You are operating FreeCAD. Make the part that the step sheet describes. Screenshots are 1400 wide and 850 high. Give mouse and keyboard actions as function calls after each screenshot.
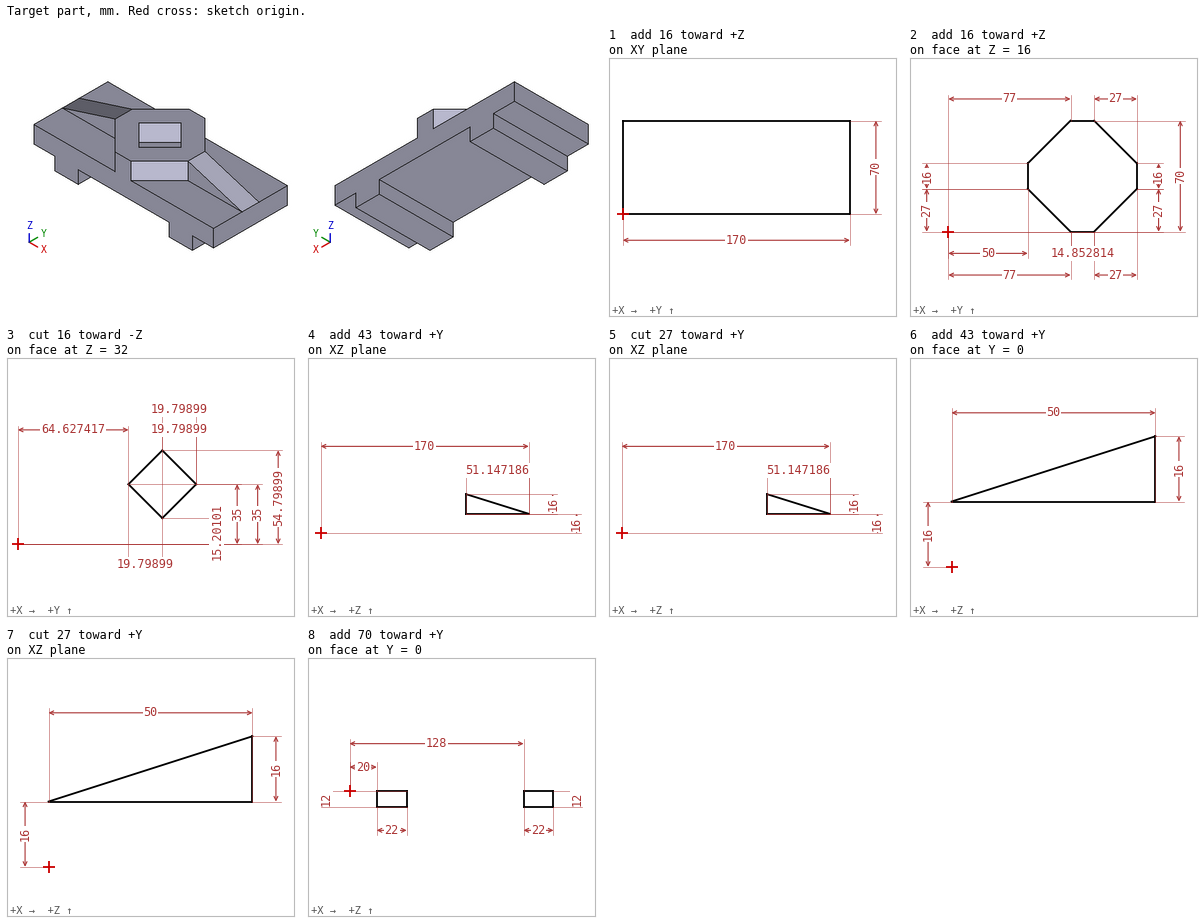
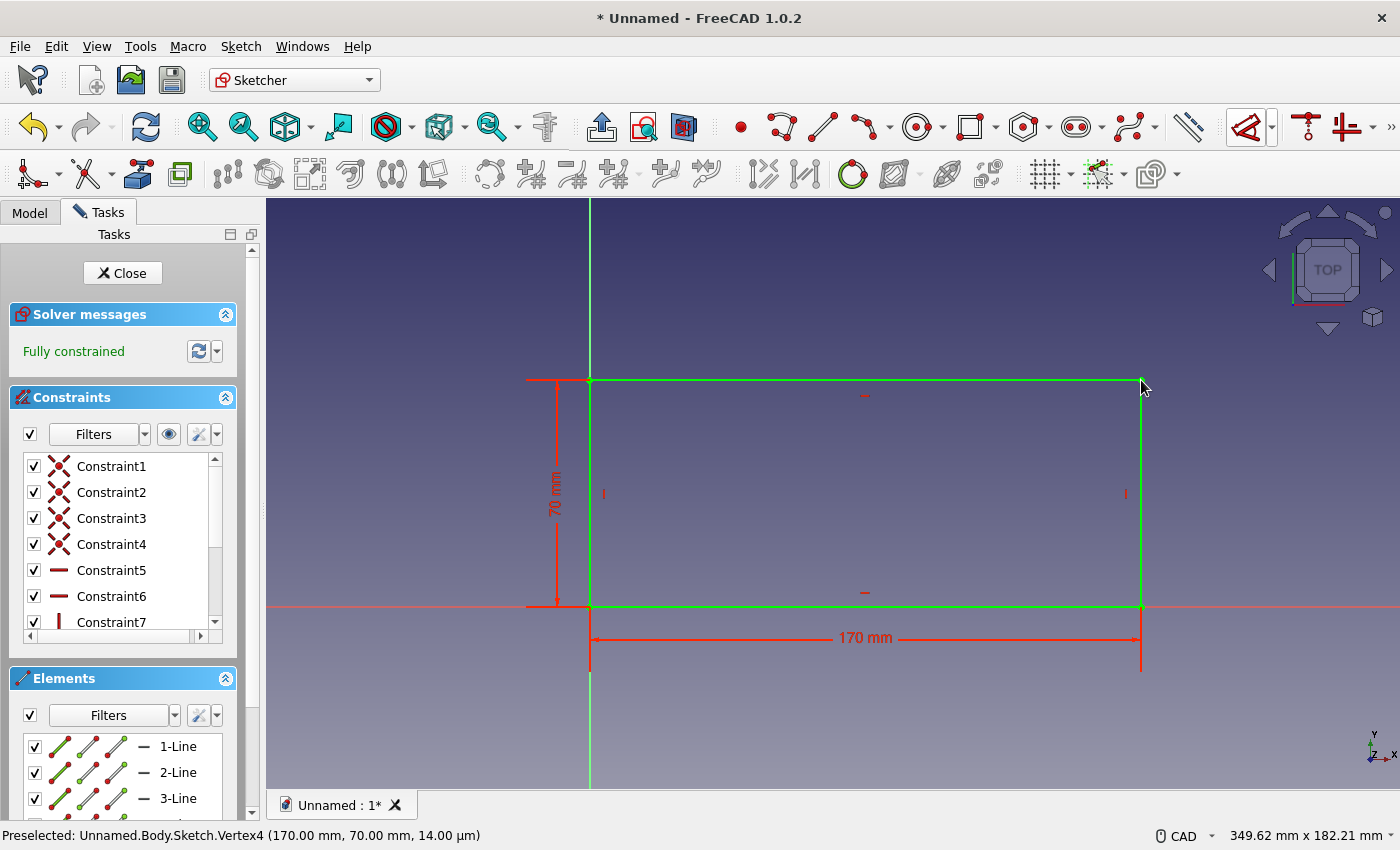
click(123, 273)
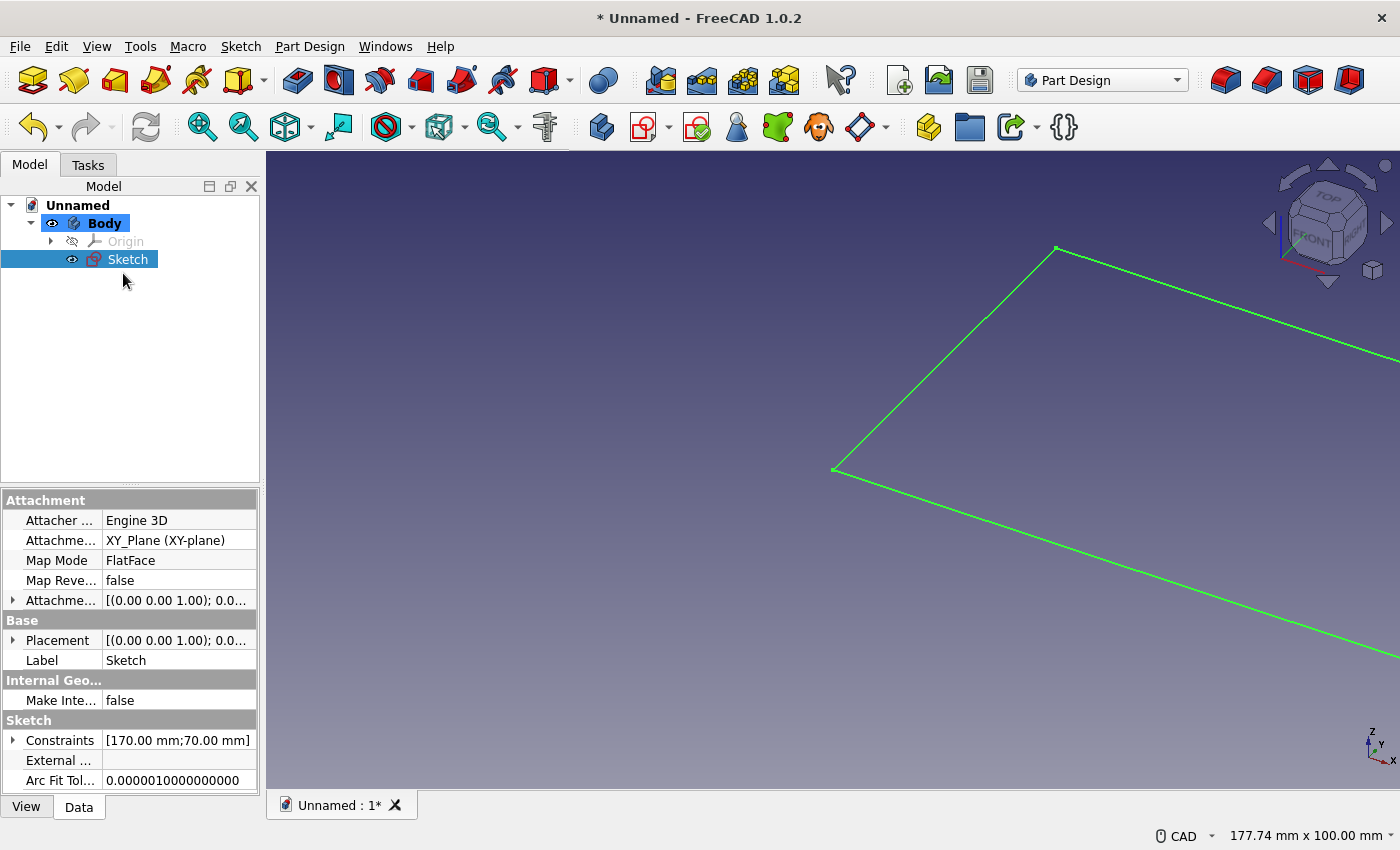
click(33, 80)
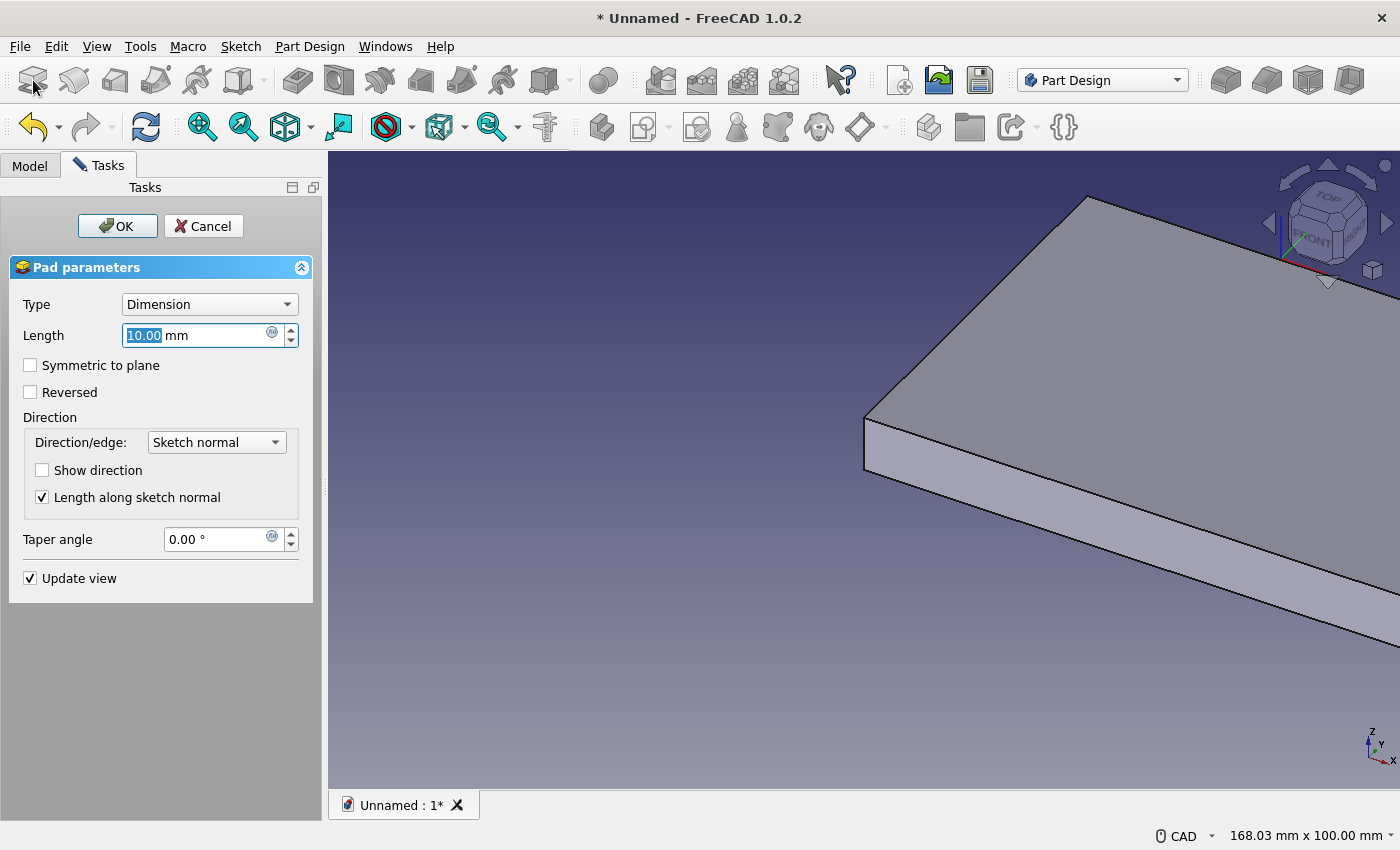
text(16)
key(Tab)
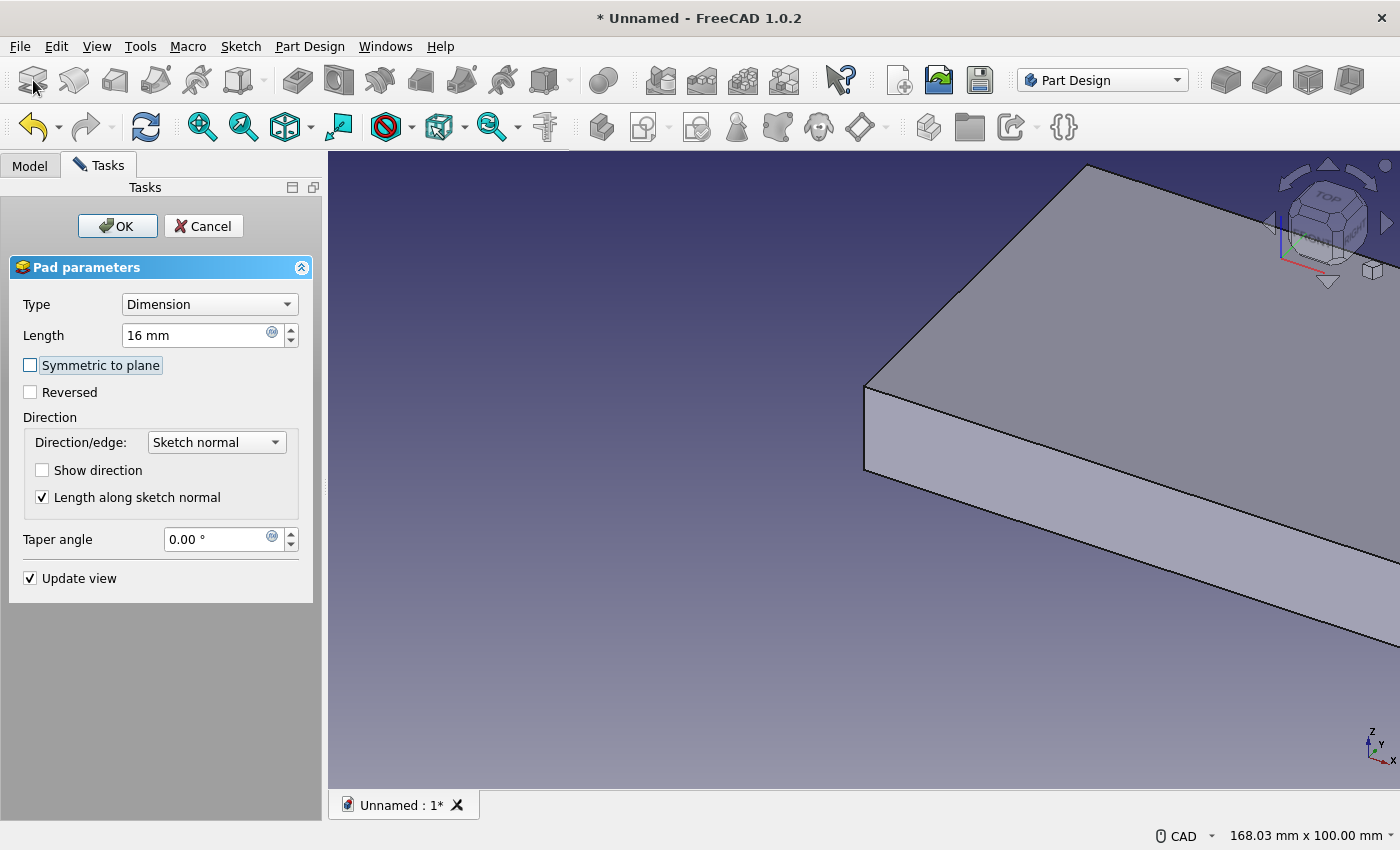
click(118, 226)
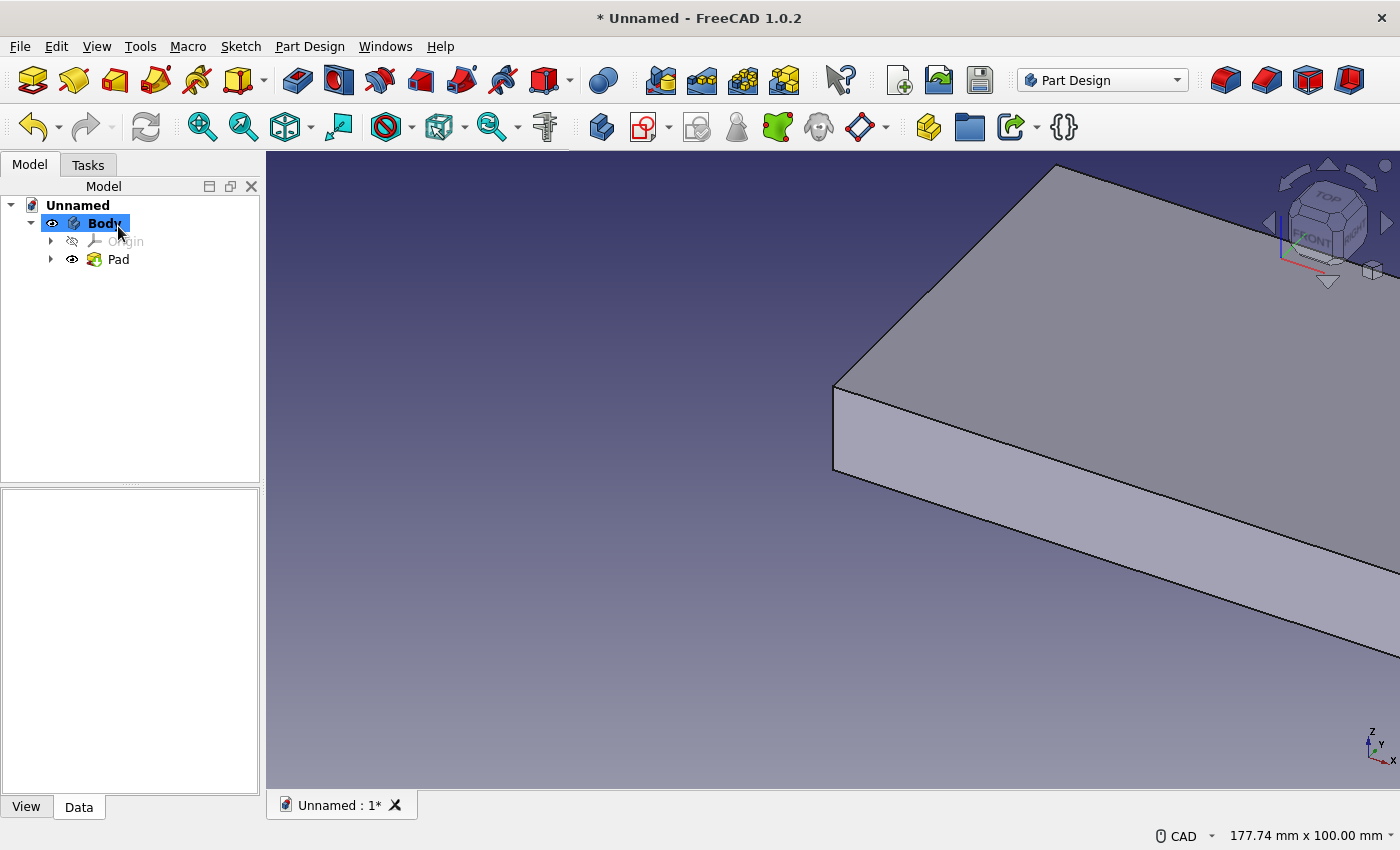
key(v)
key(f)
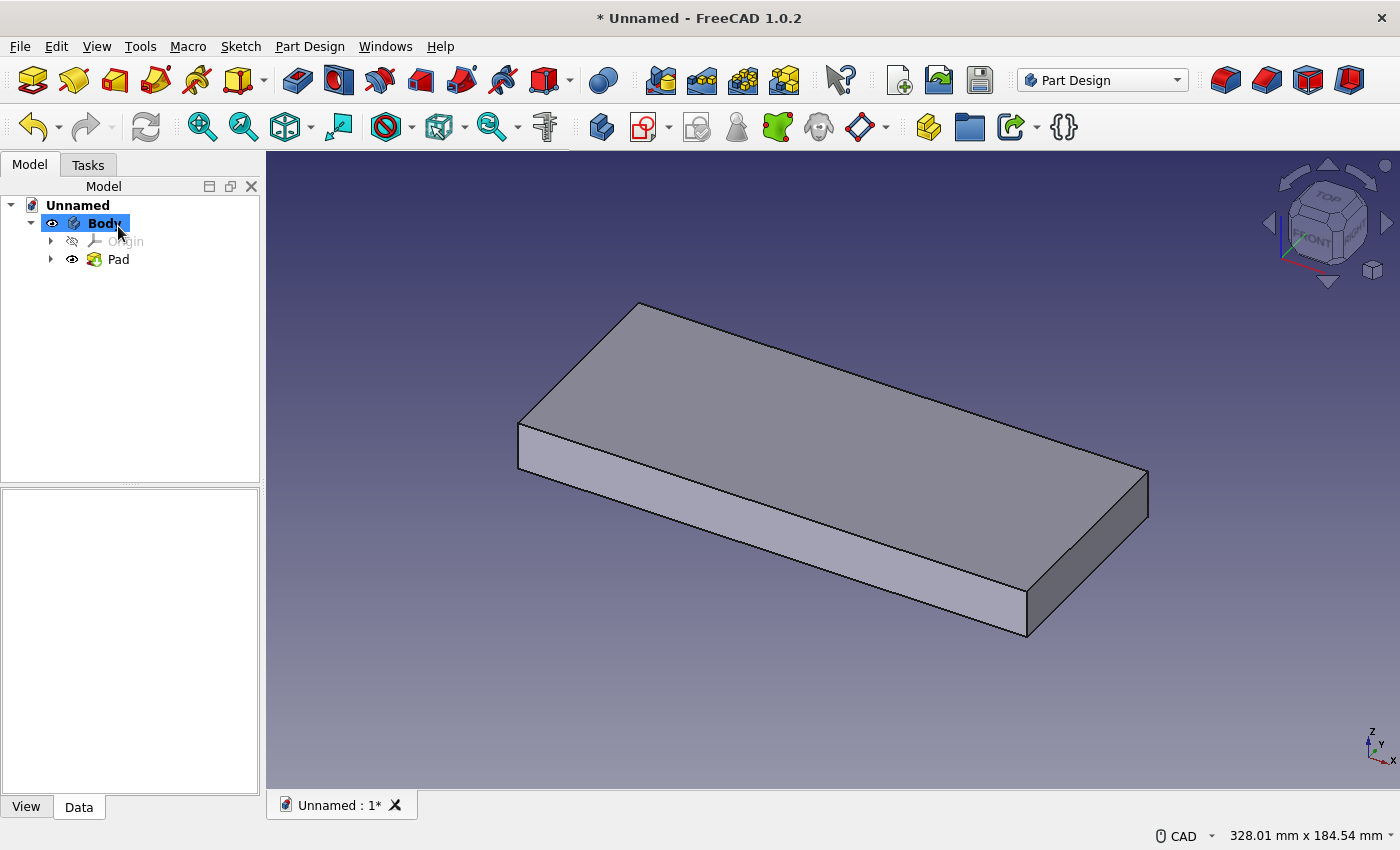
click(978, 495)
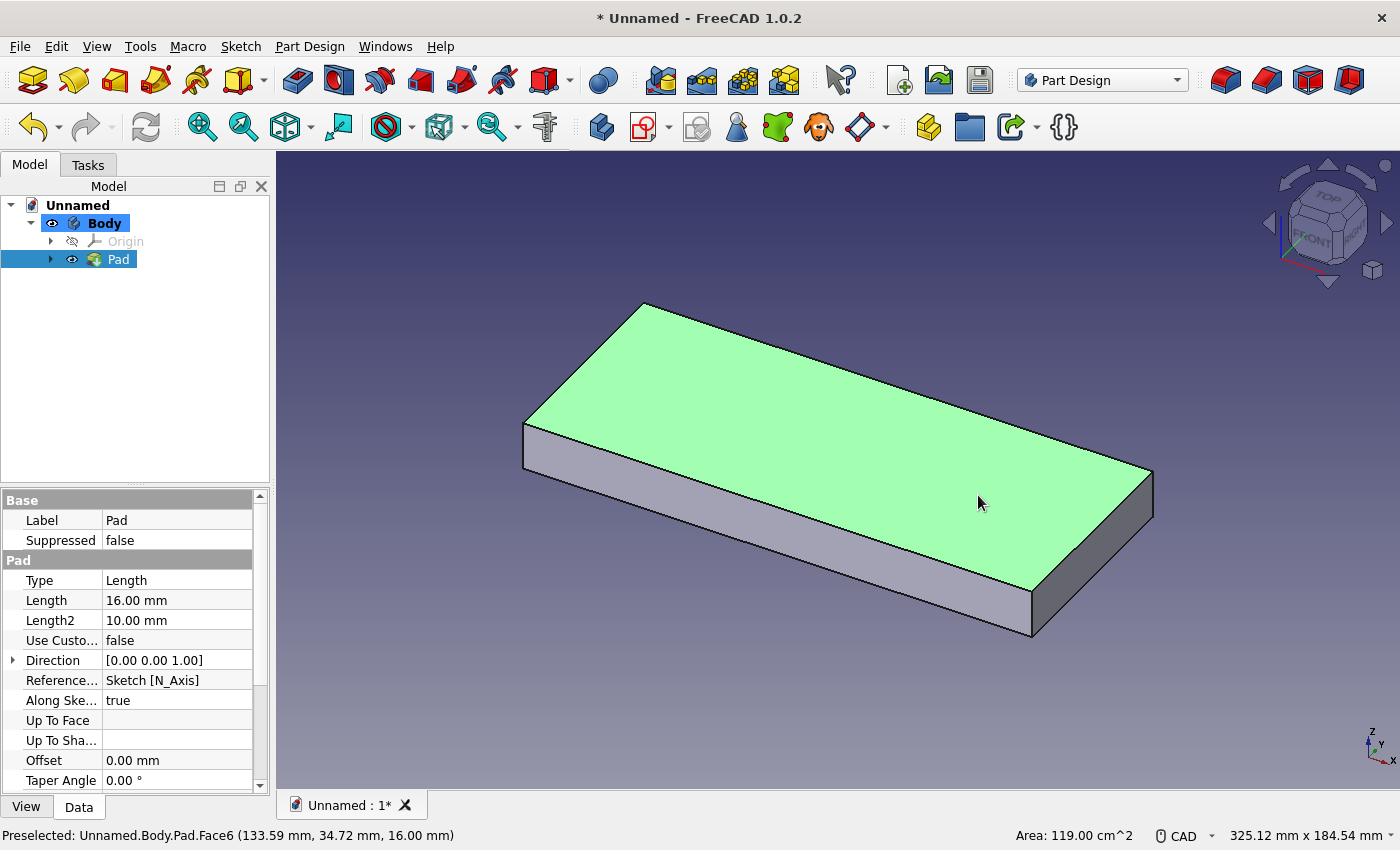
click(642, 128)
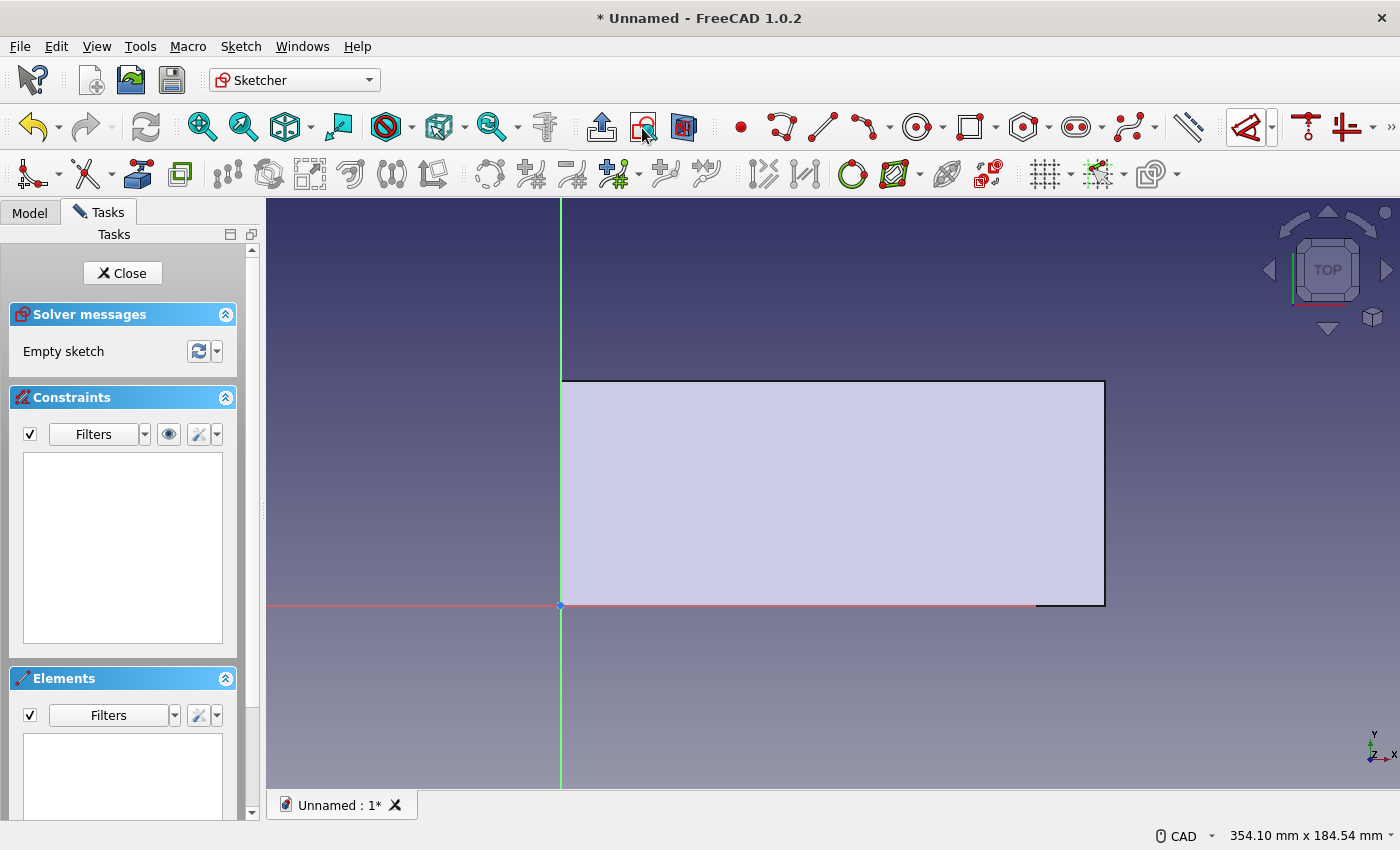
scroll(735, 494, up, 3)